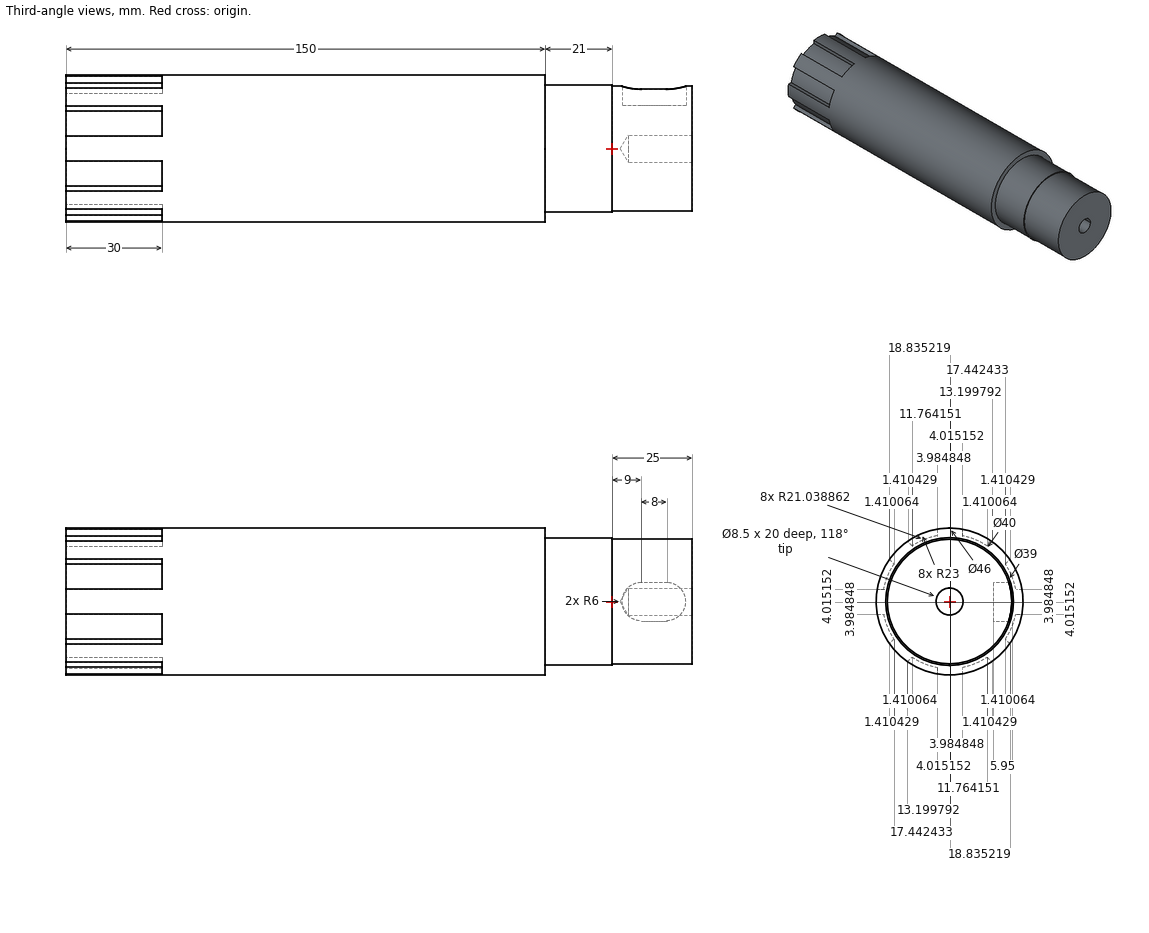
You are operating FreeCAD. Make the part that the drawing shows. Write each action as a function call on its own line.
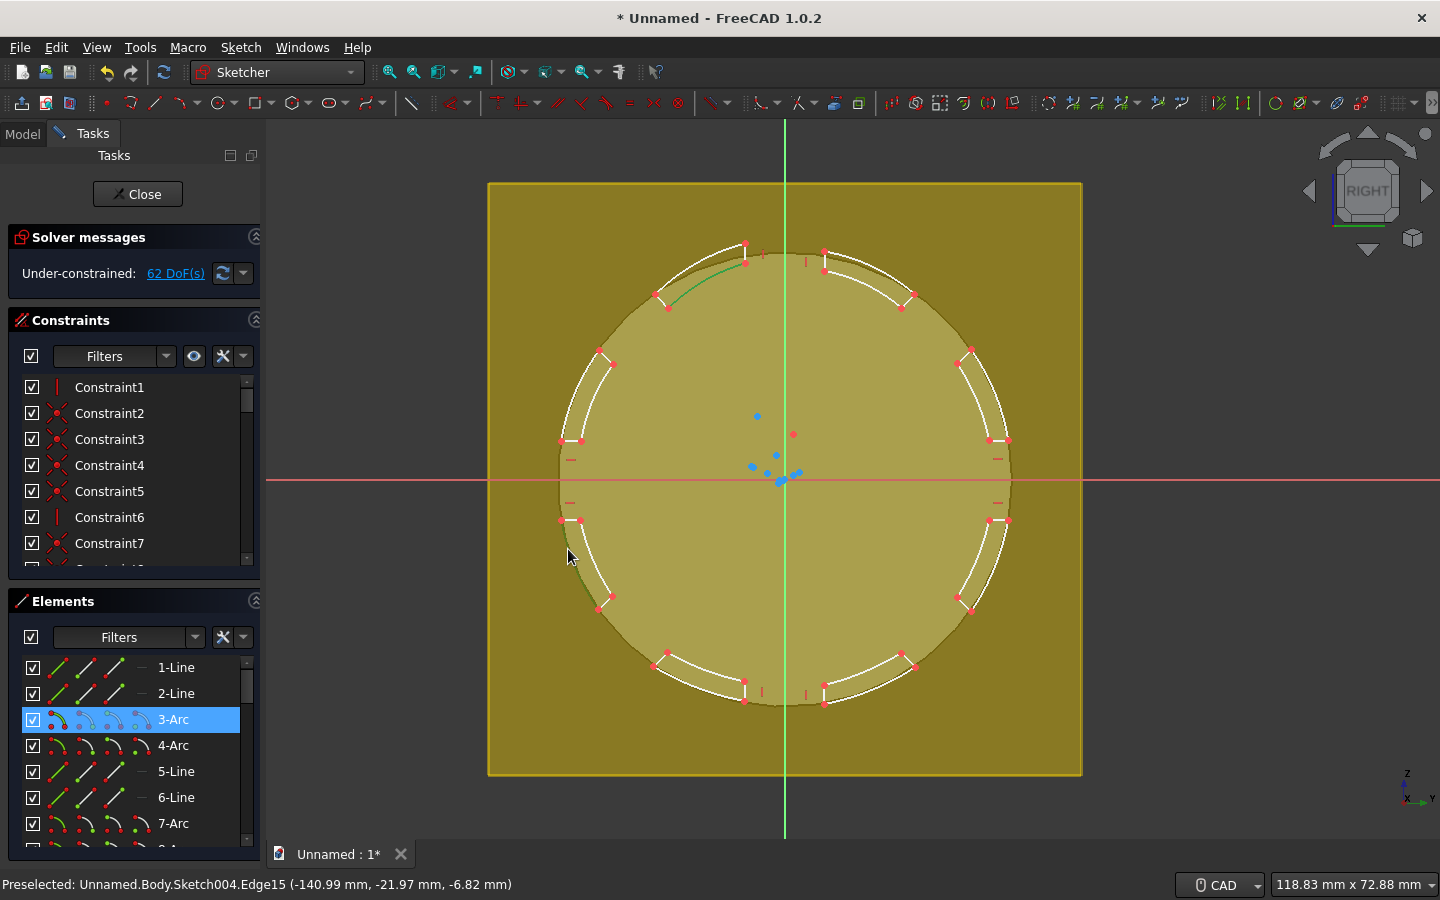
click(498, 104)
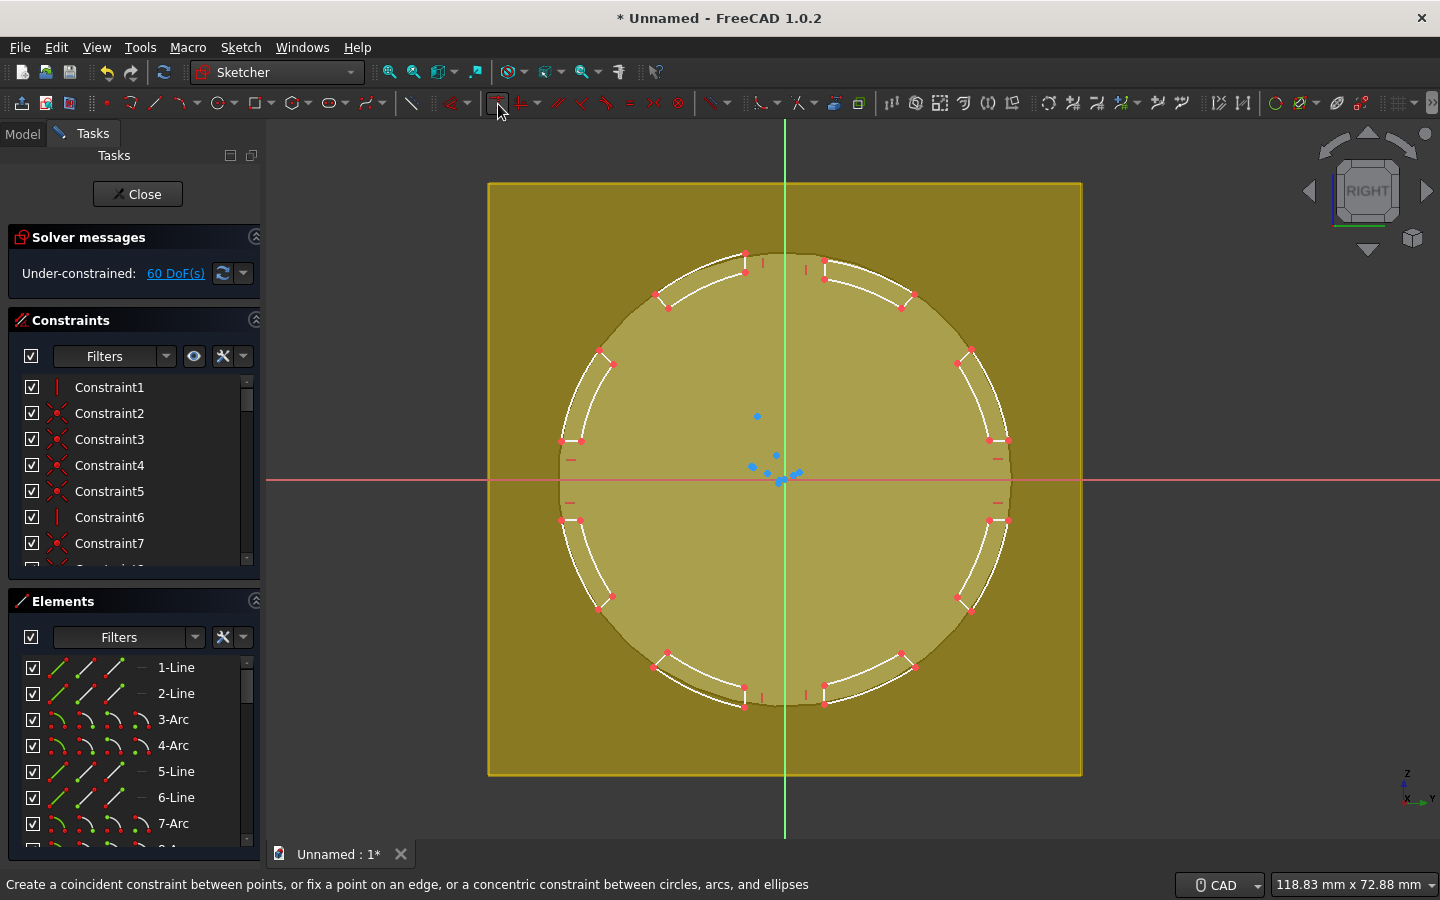
click(721, 280)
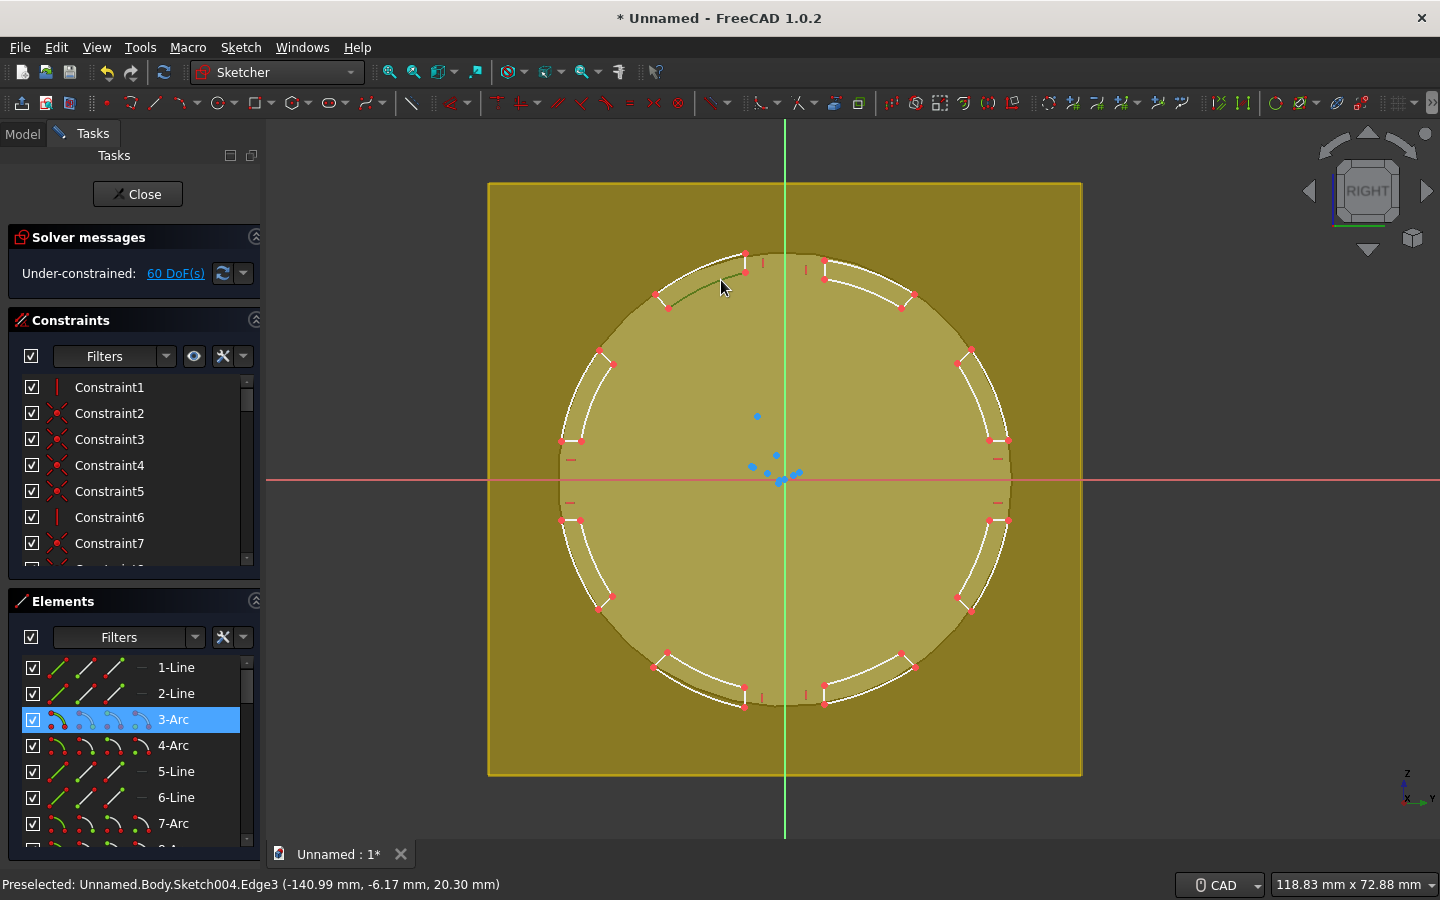
click(587, 544)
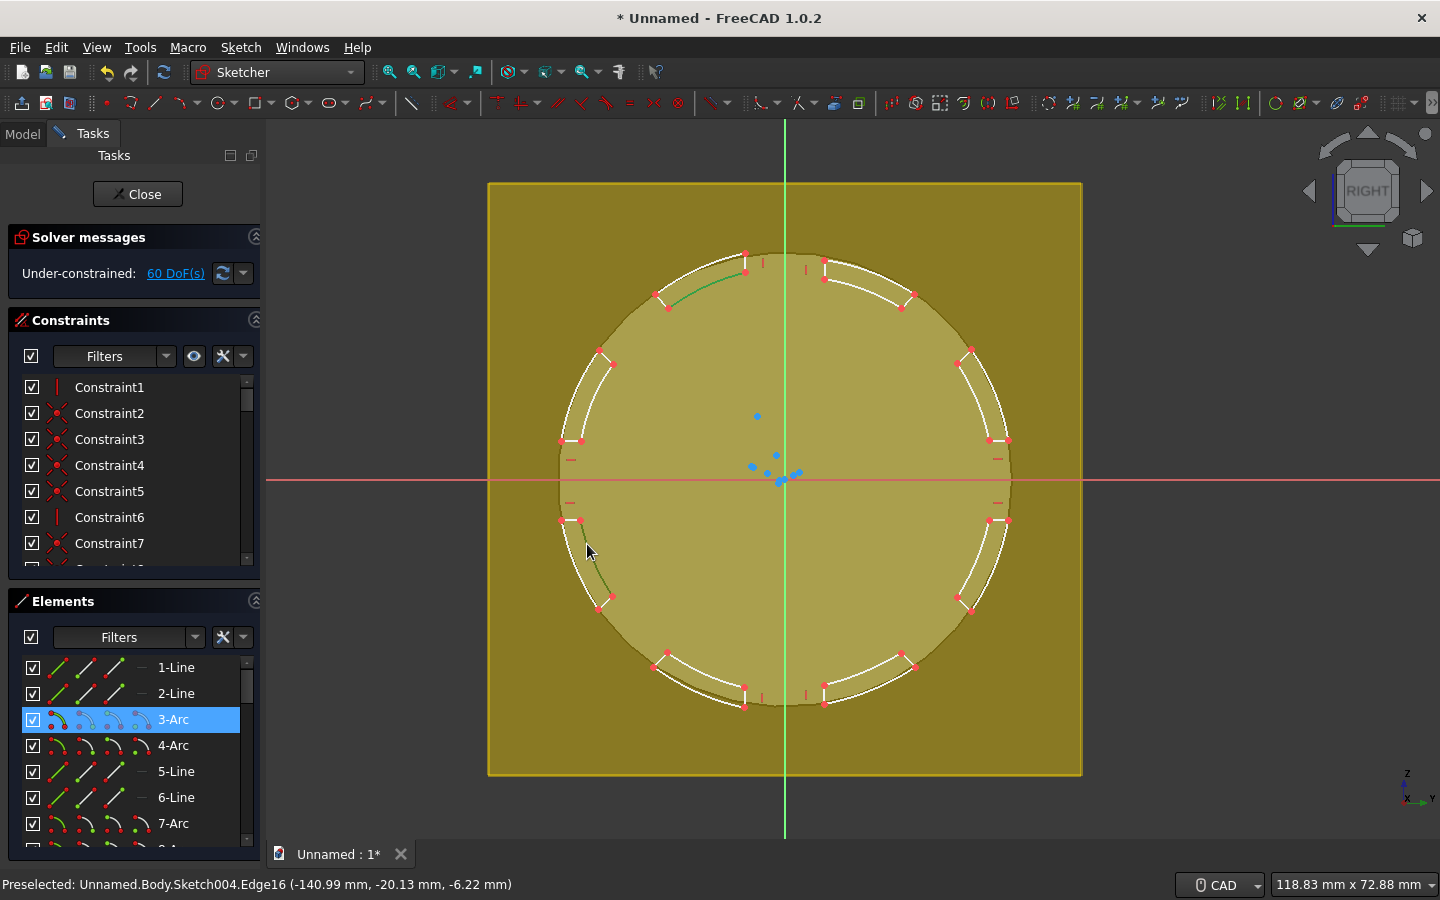
click(498, 104)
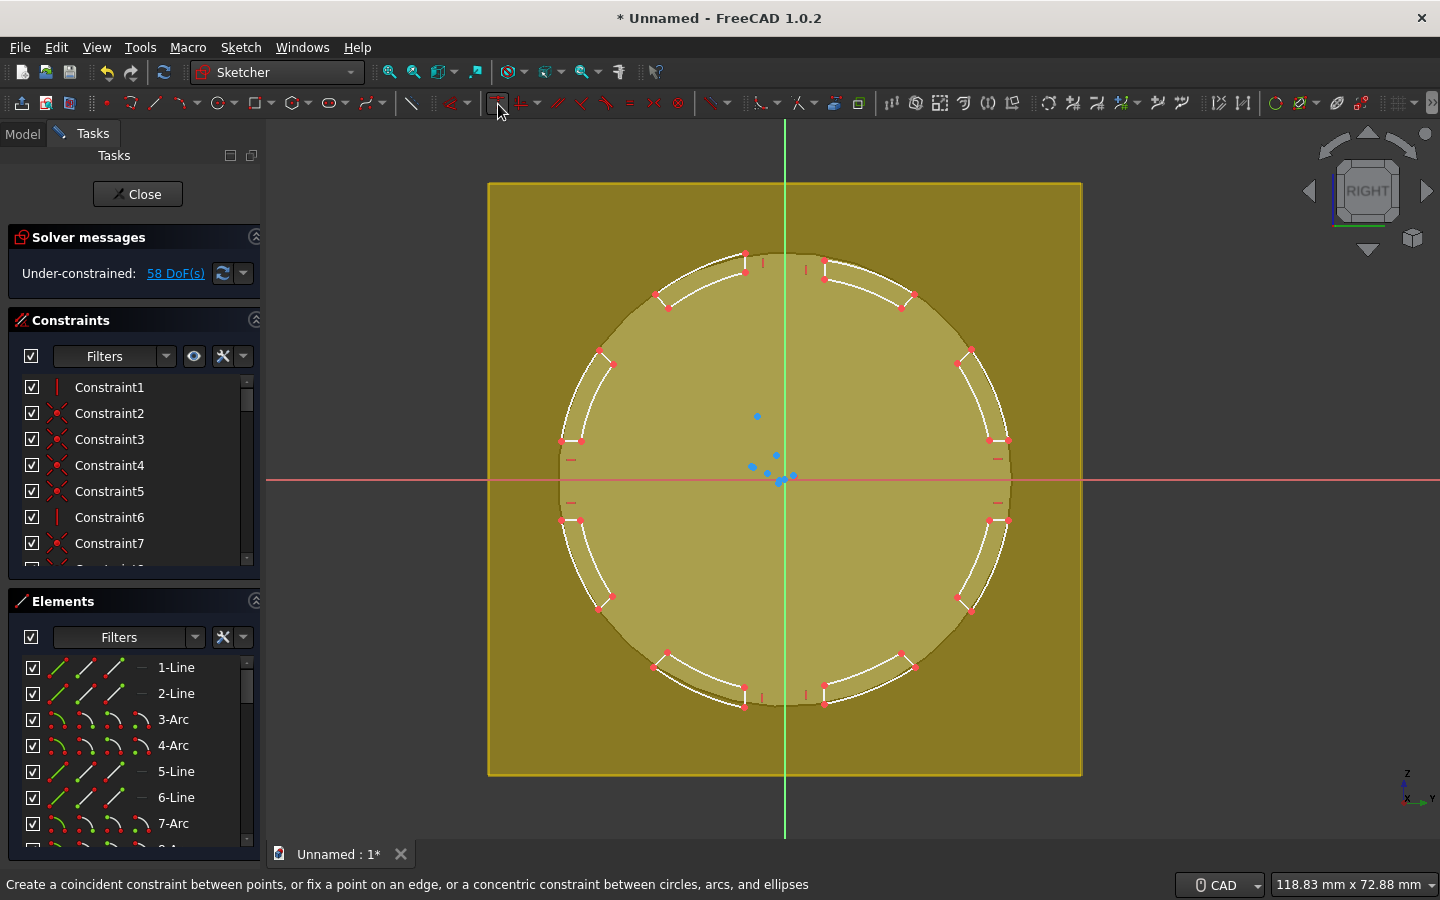
click(721, 280)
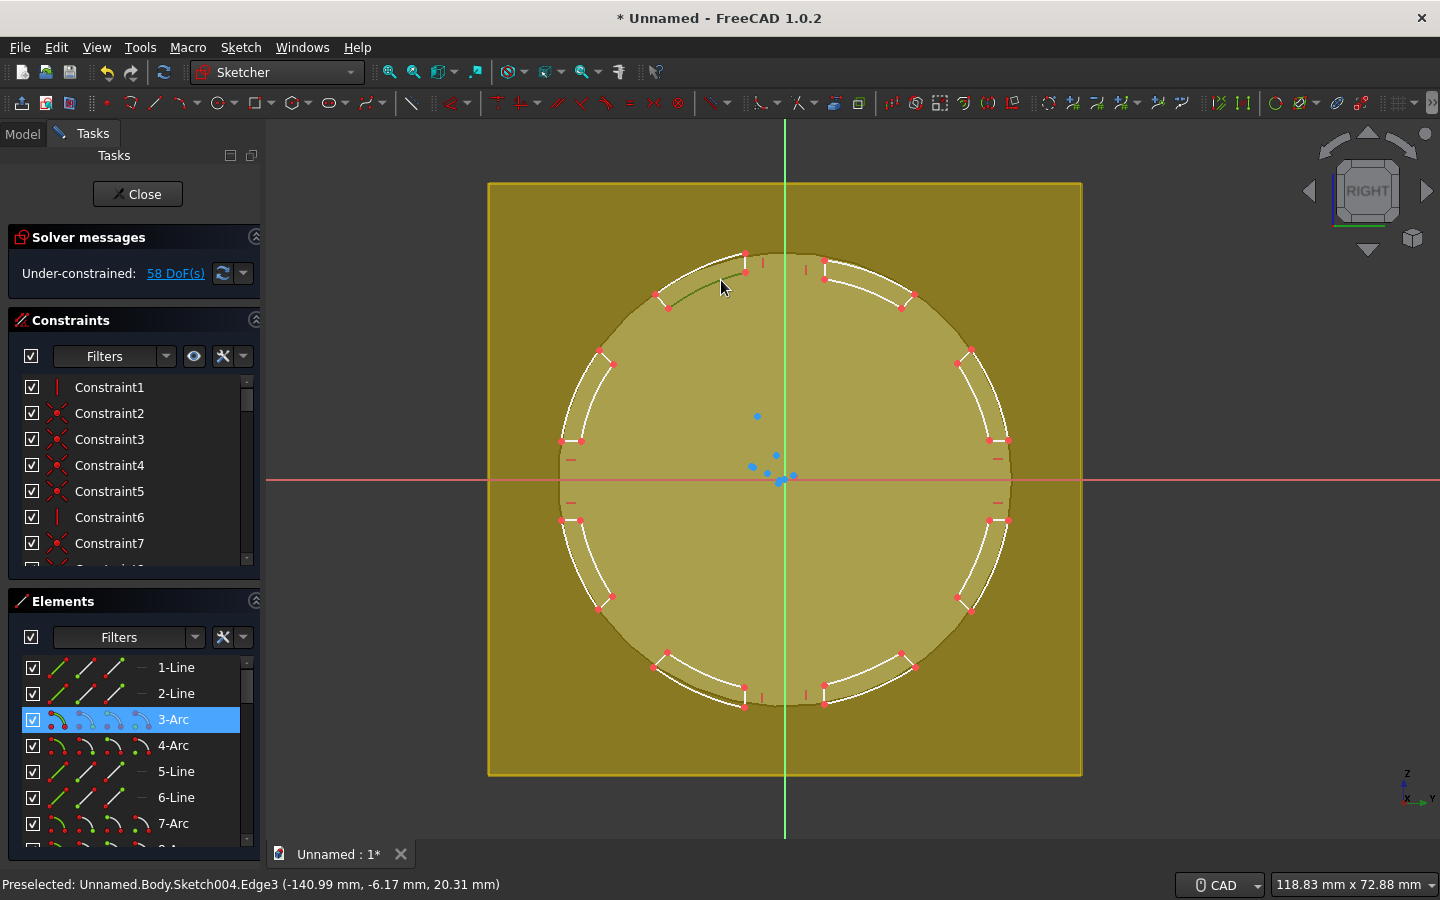
click(600, 386)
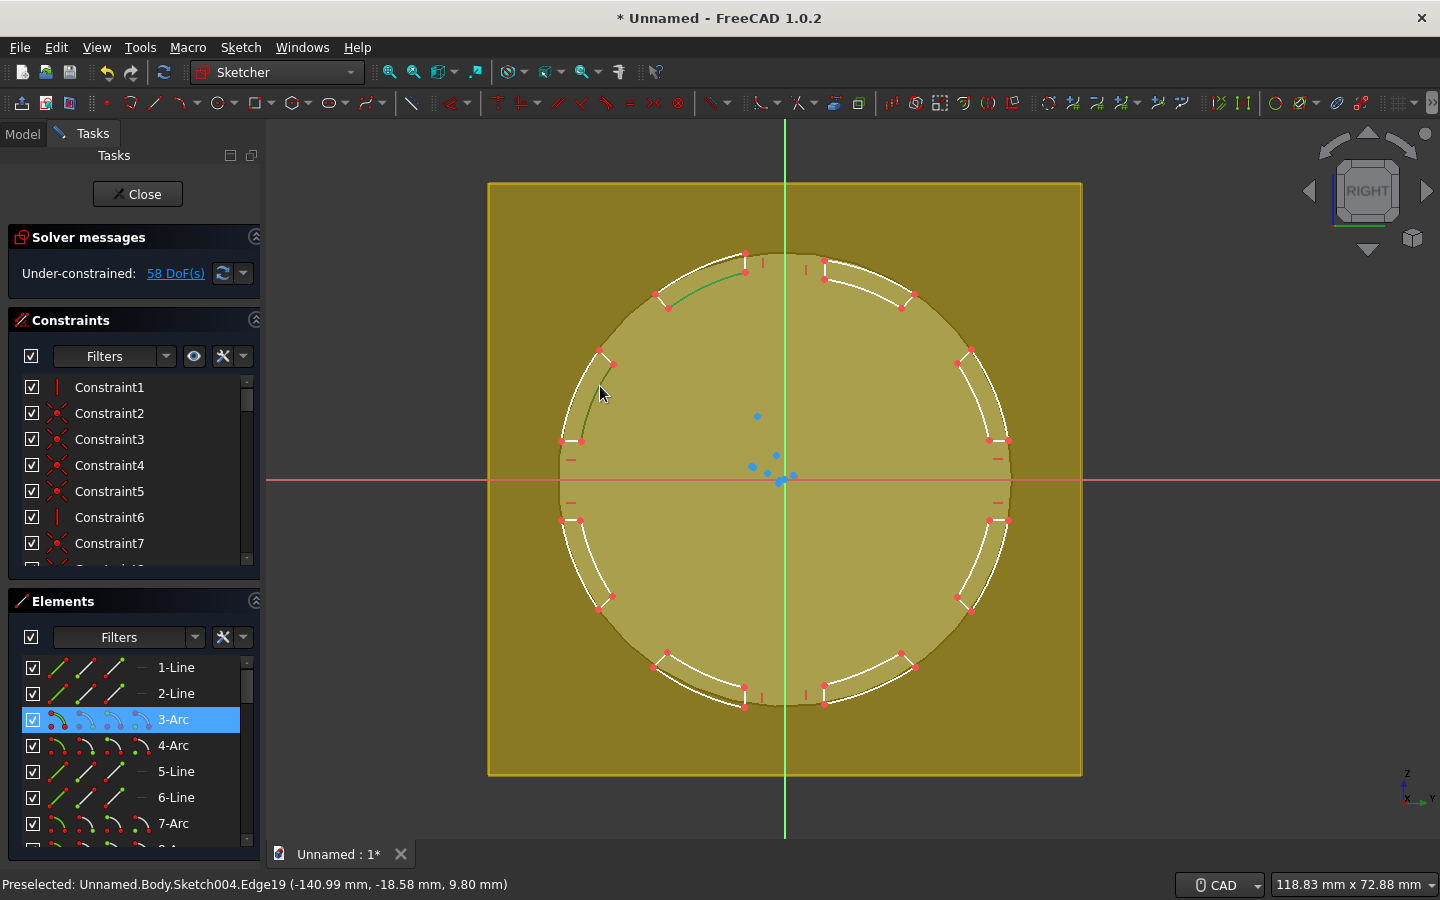
click(498, 104)